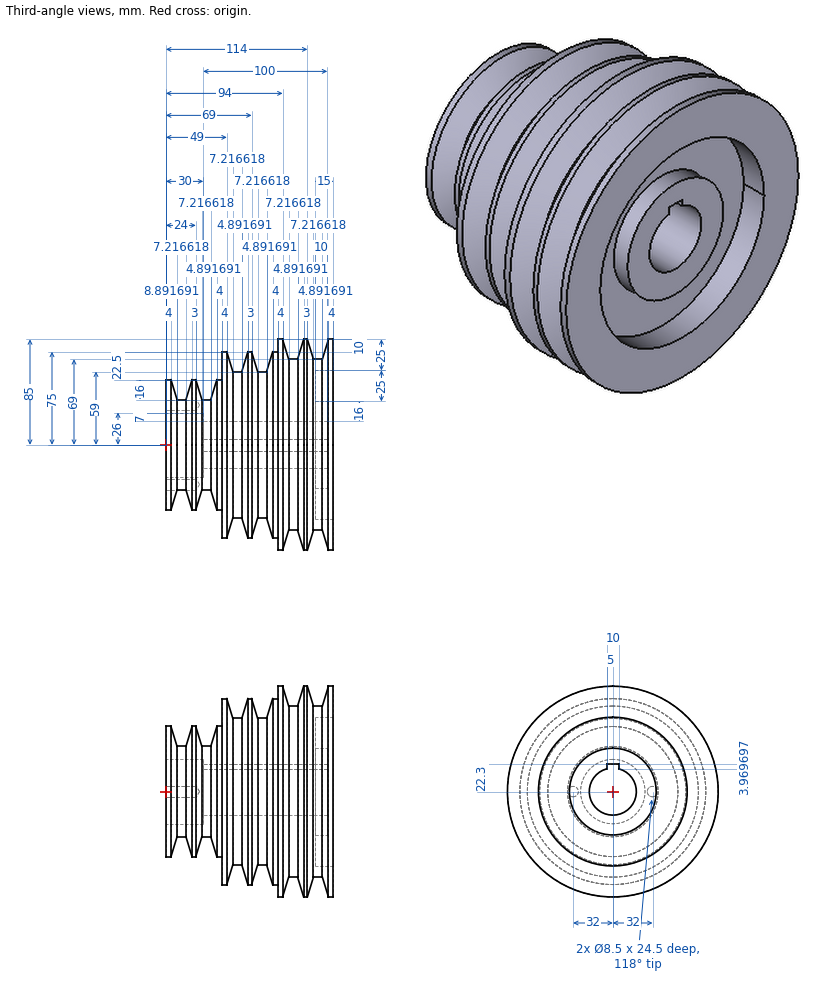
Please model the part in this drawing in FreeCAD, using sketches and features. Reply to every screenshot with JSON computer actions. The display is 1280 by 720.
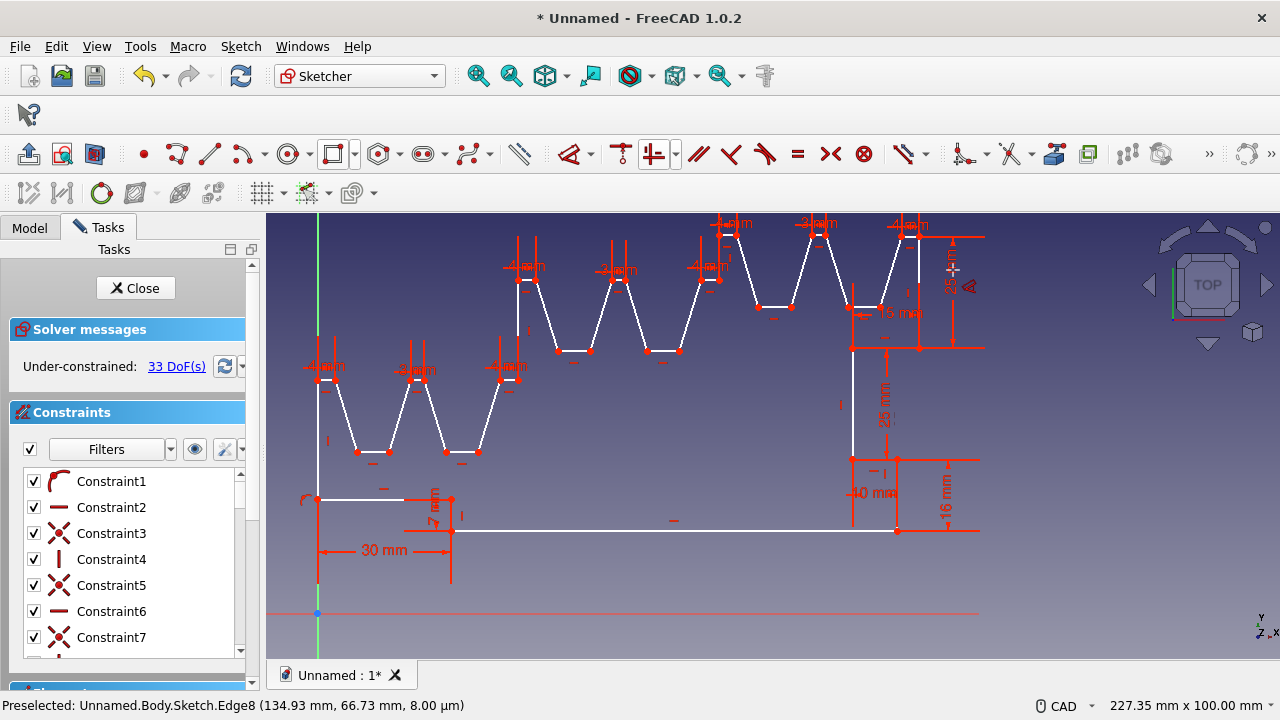
{"action": "left_click", "coordinate": [719, 249]}
{"action": "left_click", "coordinate": [685, 247]}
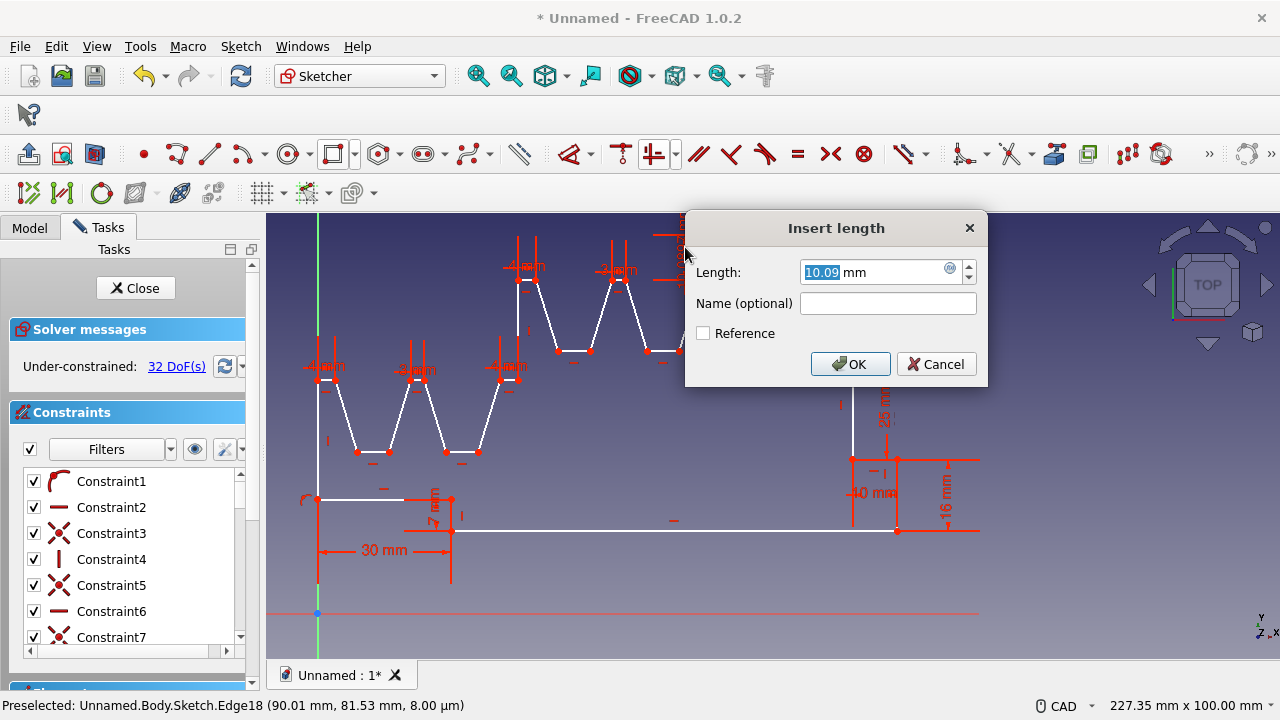
{"action": "type", "text": "10"}
{"action": "key", "text": "Return"}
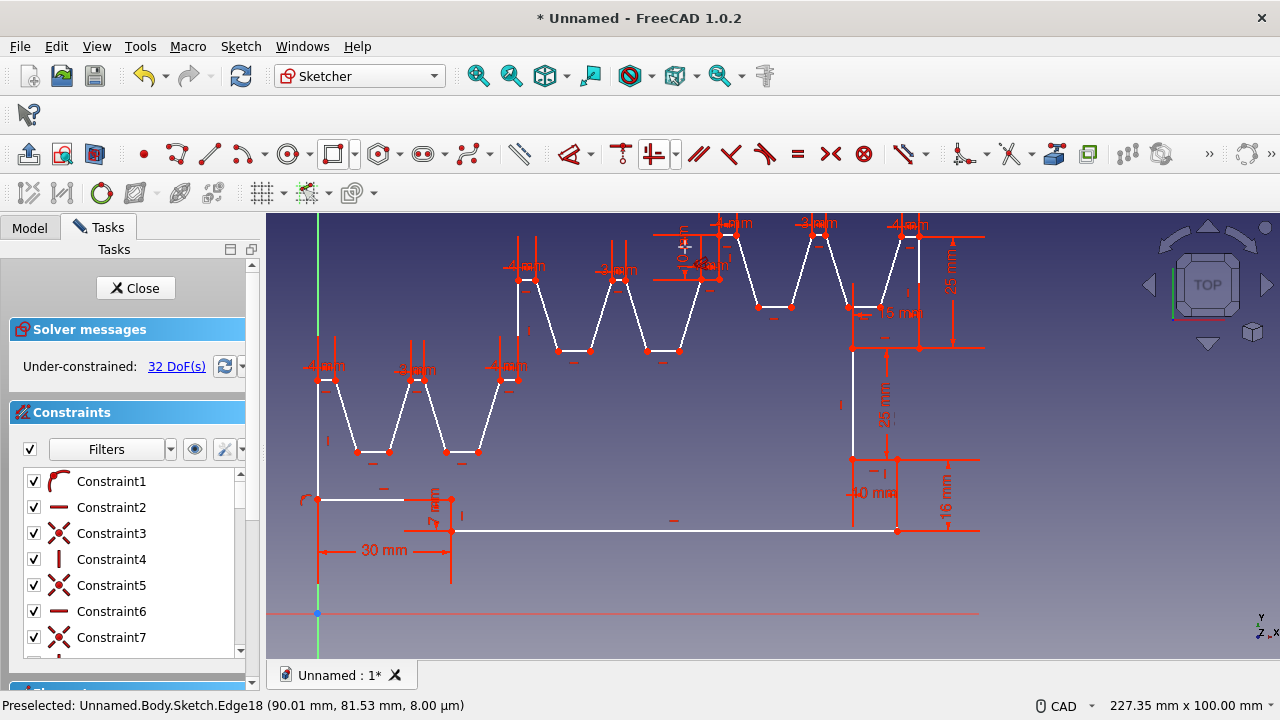
{"action": "left_click", "coordinate": [585, 531]}
{"action": "left_click", "coordinate": [674, 565]}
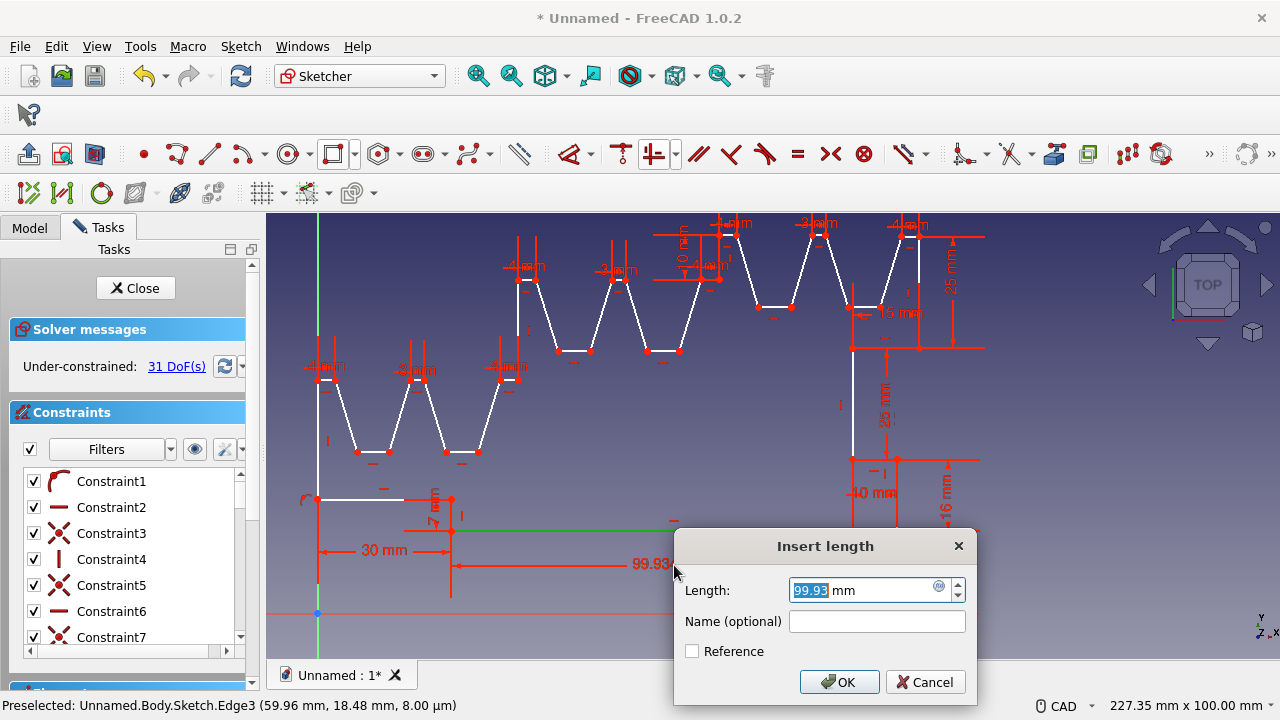
{"action": "type", "text": "100"}
{"action": "key", "text": "Return"}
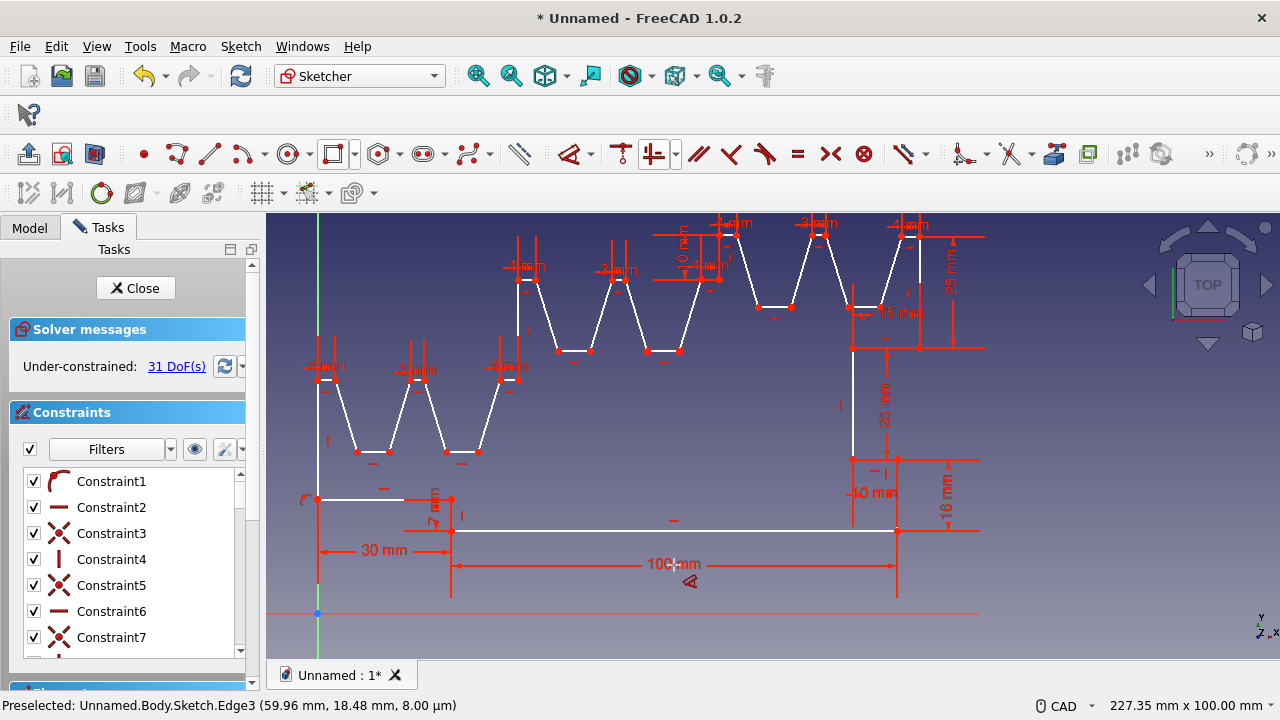
{"action": "left_click", "coordinate": [318, 500]}
{"action": "left_click", "coordinate": [352, 583]}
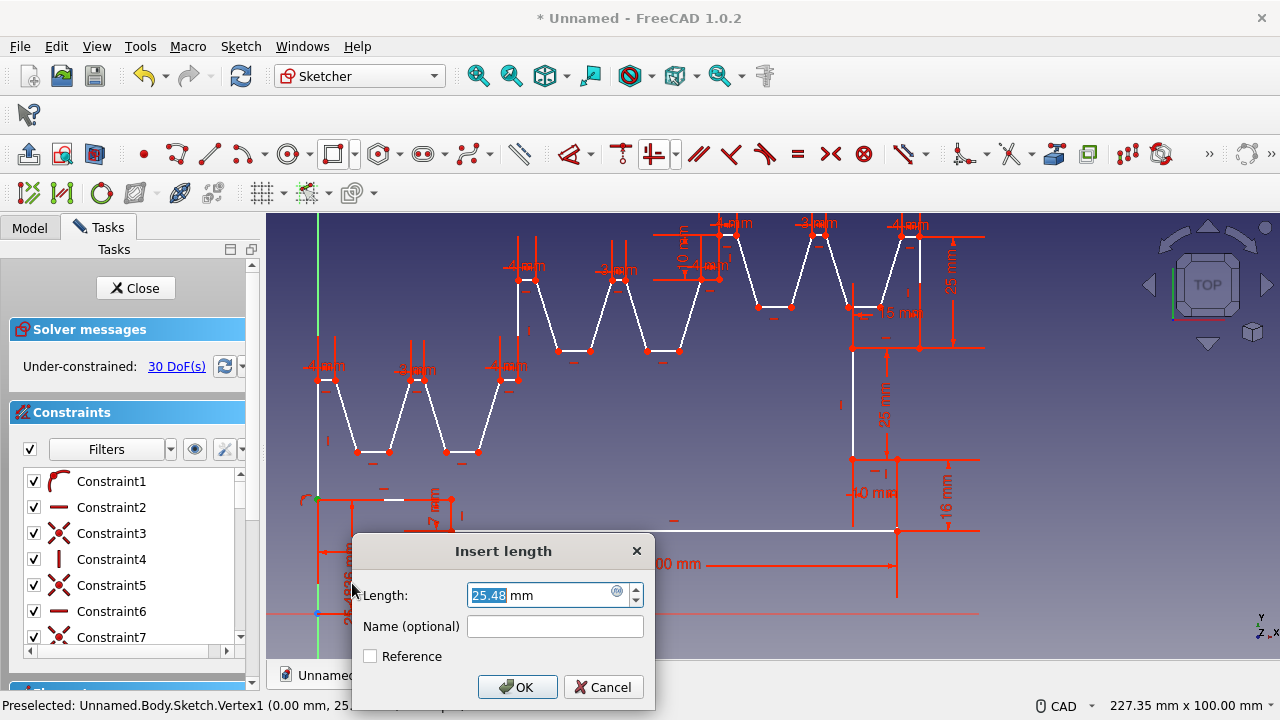
{"action": "type", "text": "26"}
{"action": "key", "text": "Return"}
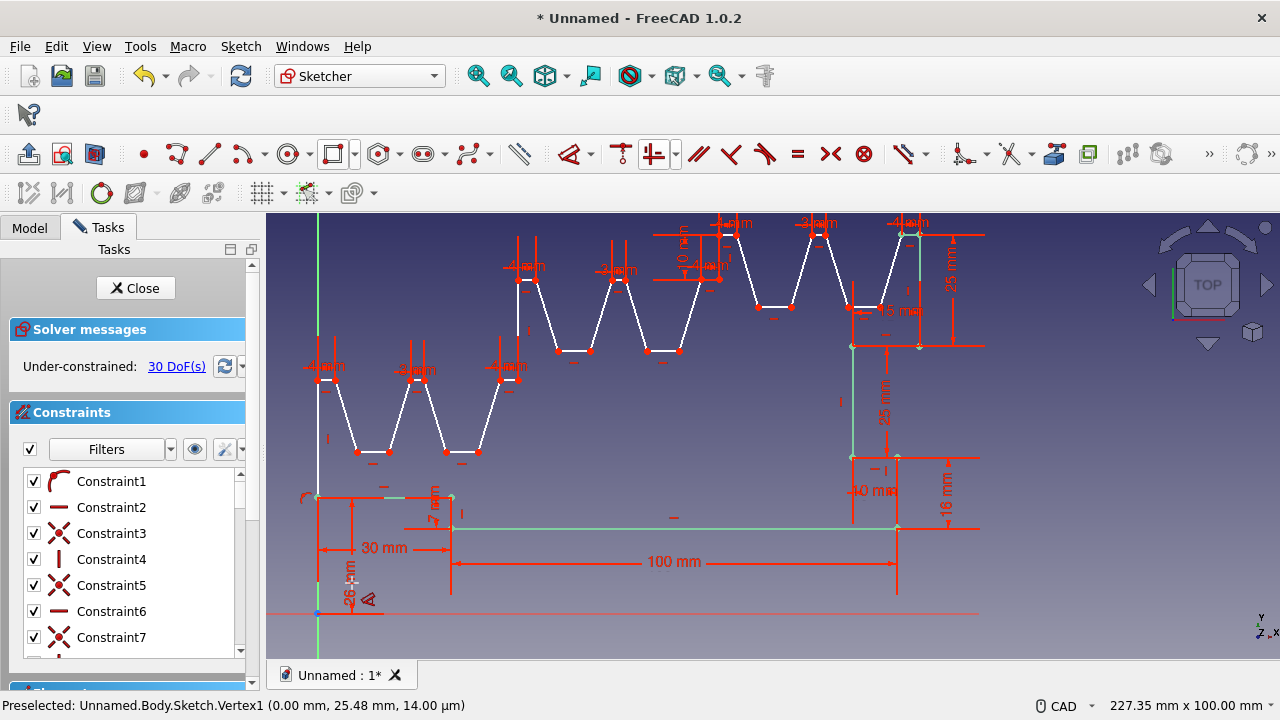
{"action": "left_click", "coordinate": [880, 307]}
{"action": "left_click", "coordinate": [914, 460]}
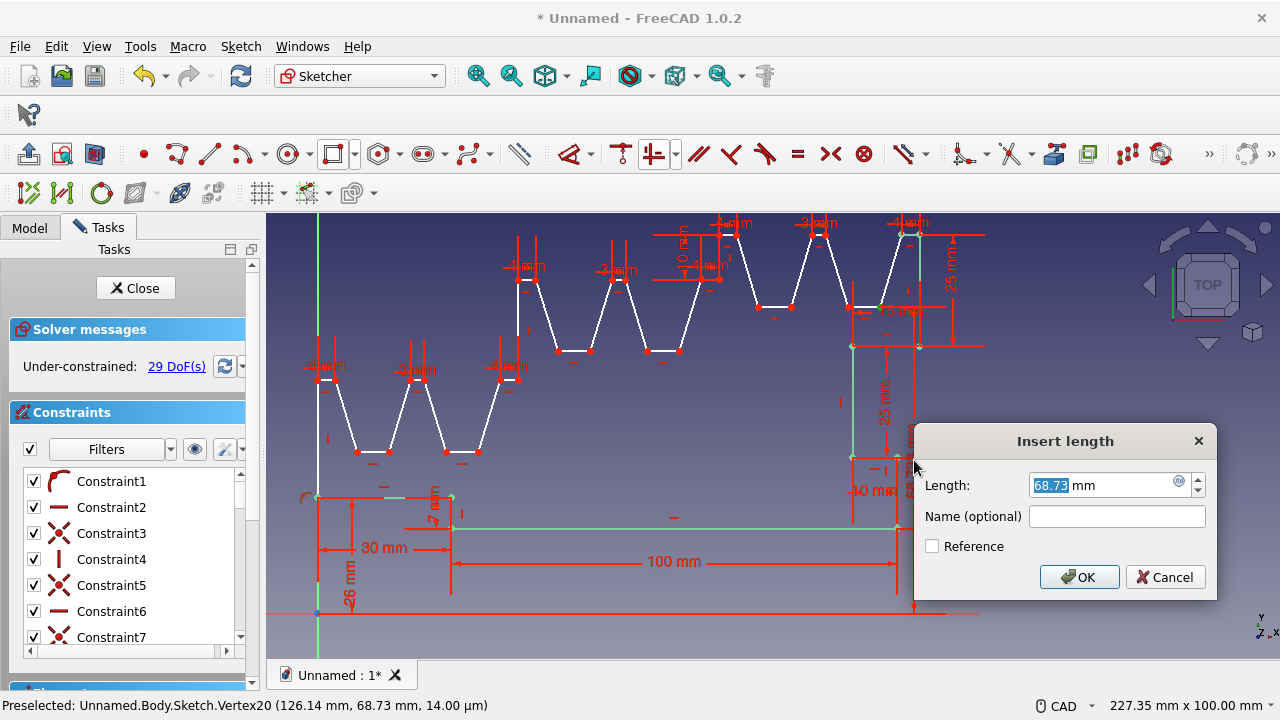
{"action": "type", "text": "69"}
{"action": "key", "text": "Return"}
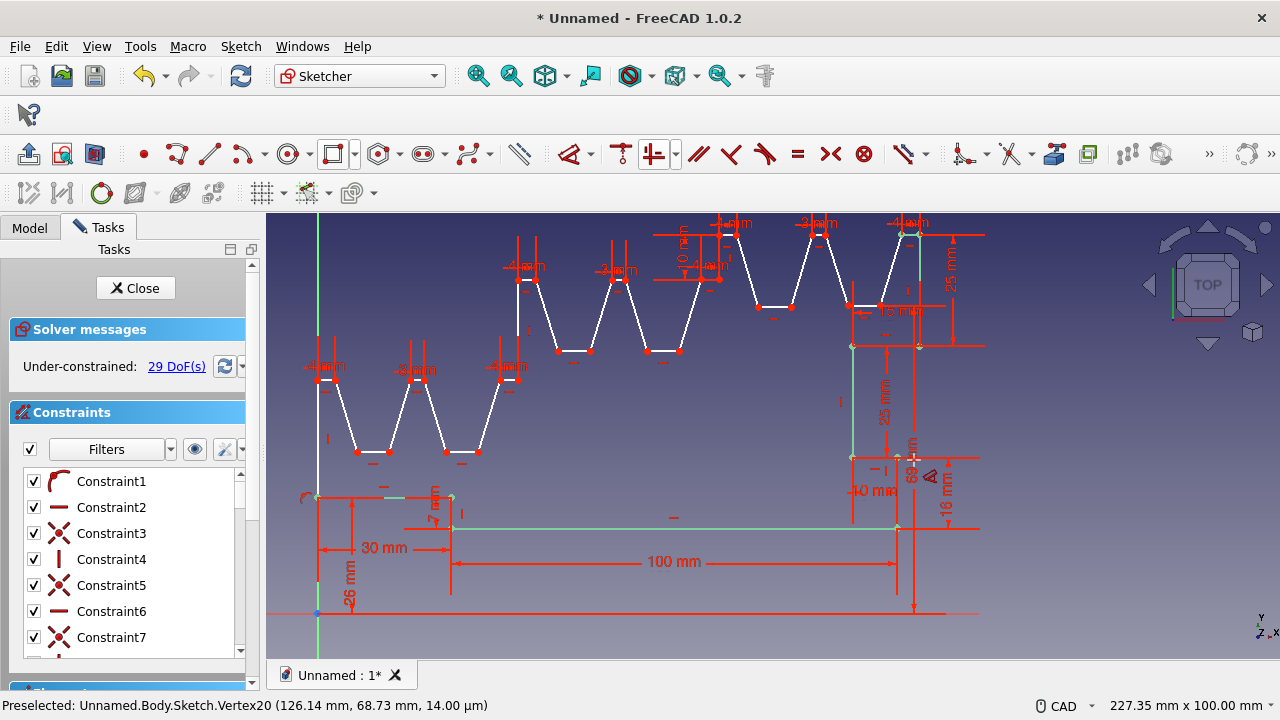
{"action": "scroll", "coordinate": [879, 460], "scroll_direction": "down", "scroll_amount": 2}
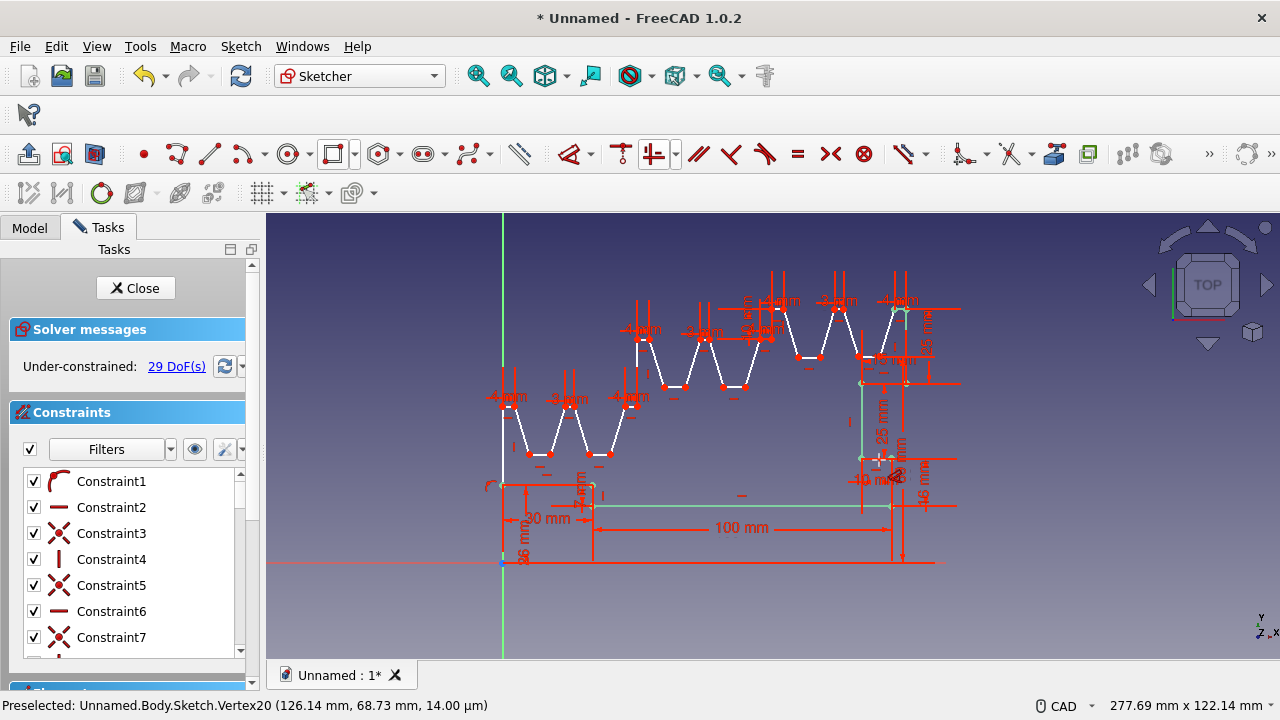
{"action": "scroll", "coordinate": [844, 309], "scroll_direction": "up", "scroll_amount": 2}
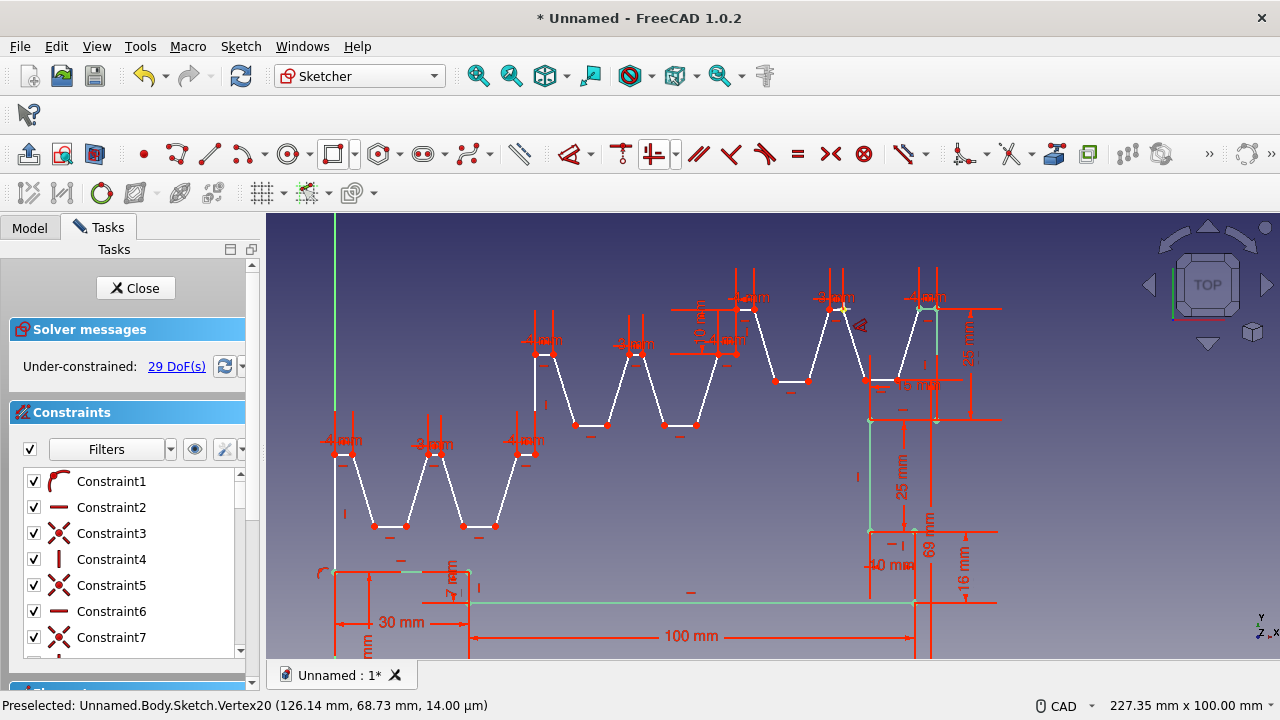
{"action": "left_click", "coordinate": [843, 310]}
{"action": "left_click", "coordinate": [301, 470]}